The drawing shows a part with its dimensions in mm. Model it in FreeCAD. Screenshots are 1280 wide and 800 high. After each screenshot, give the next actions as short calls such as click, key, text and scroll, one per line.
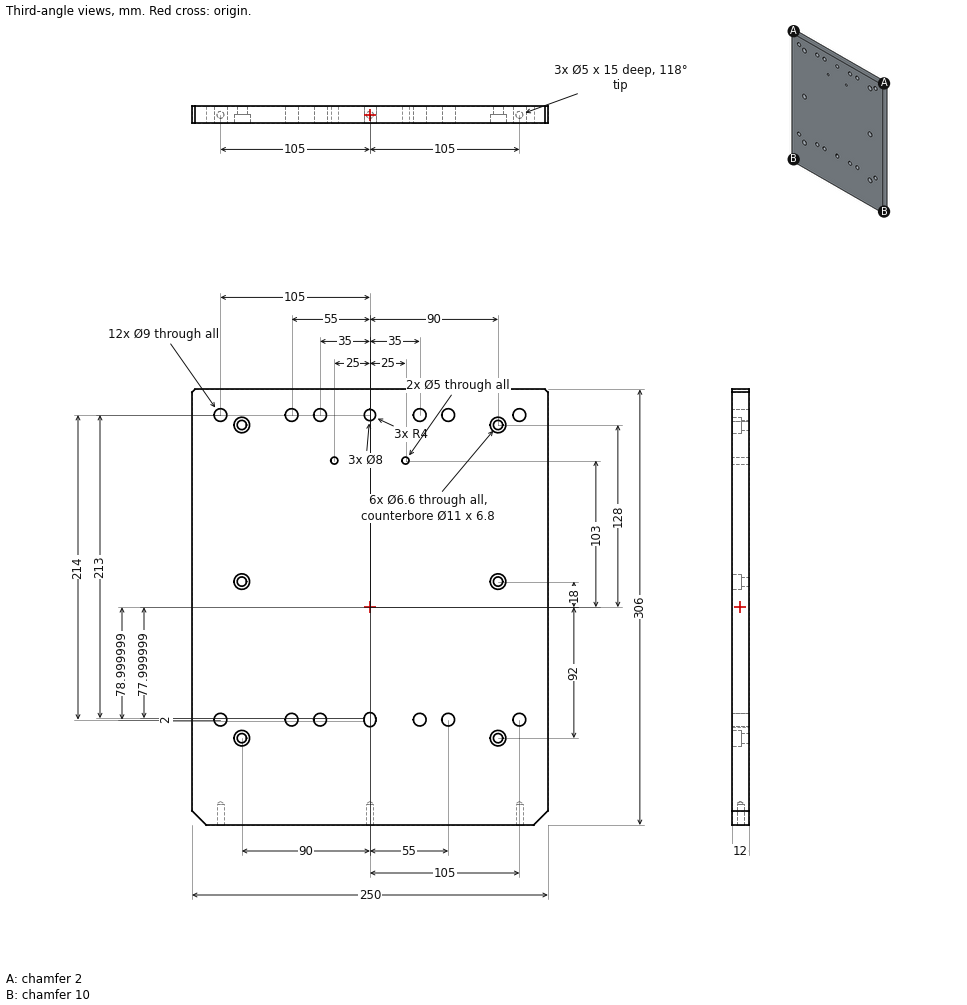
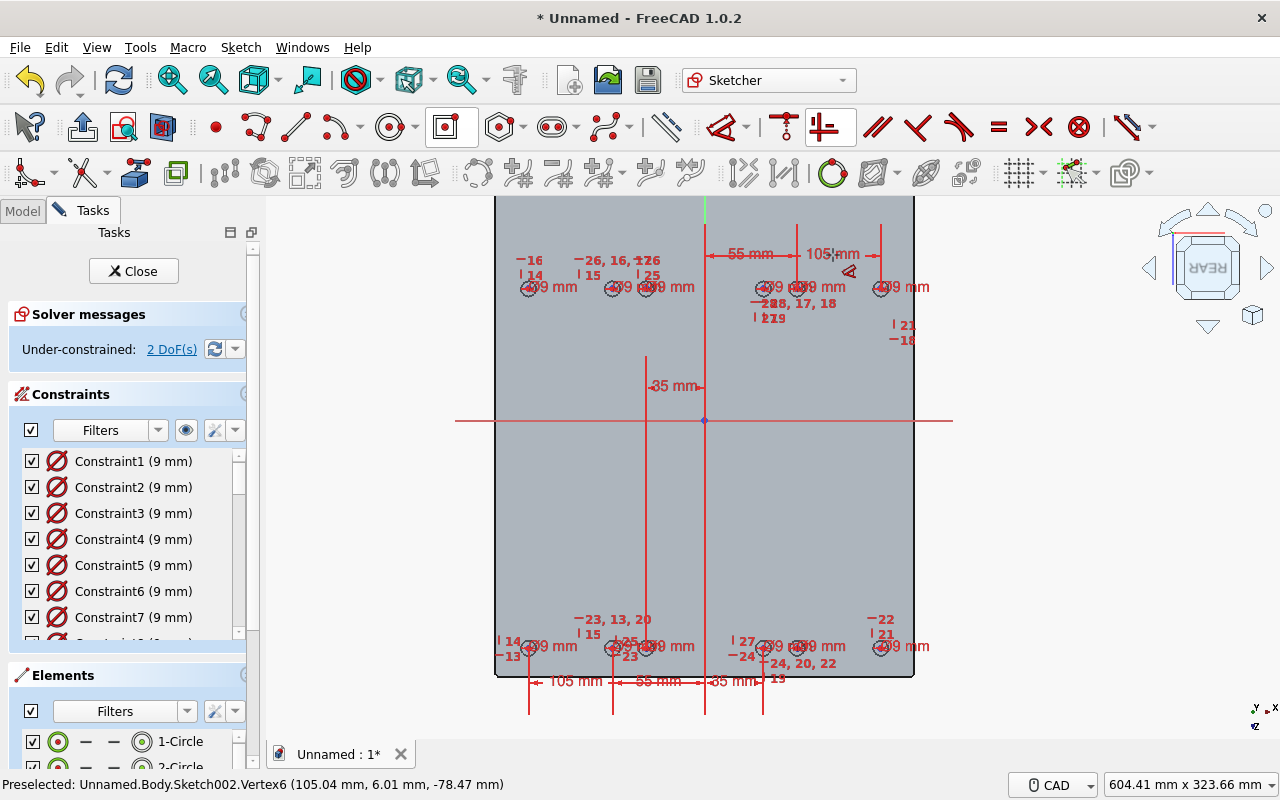
click(529, 648)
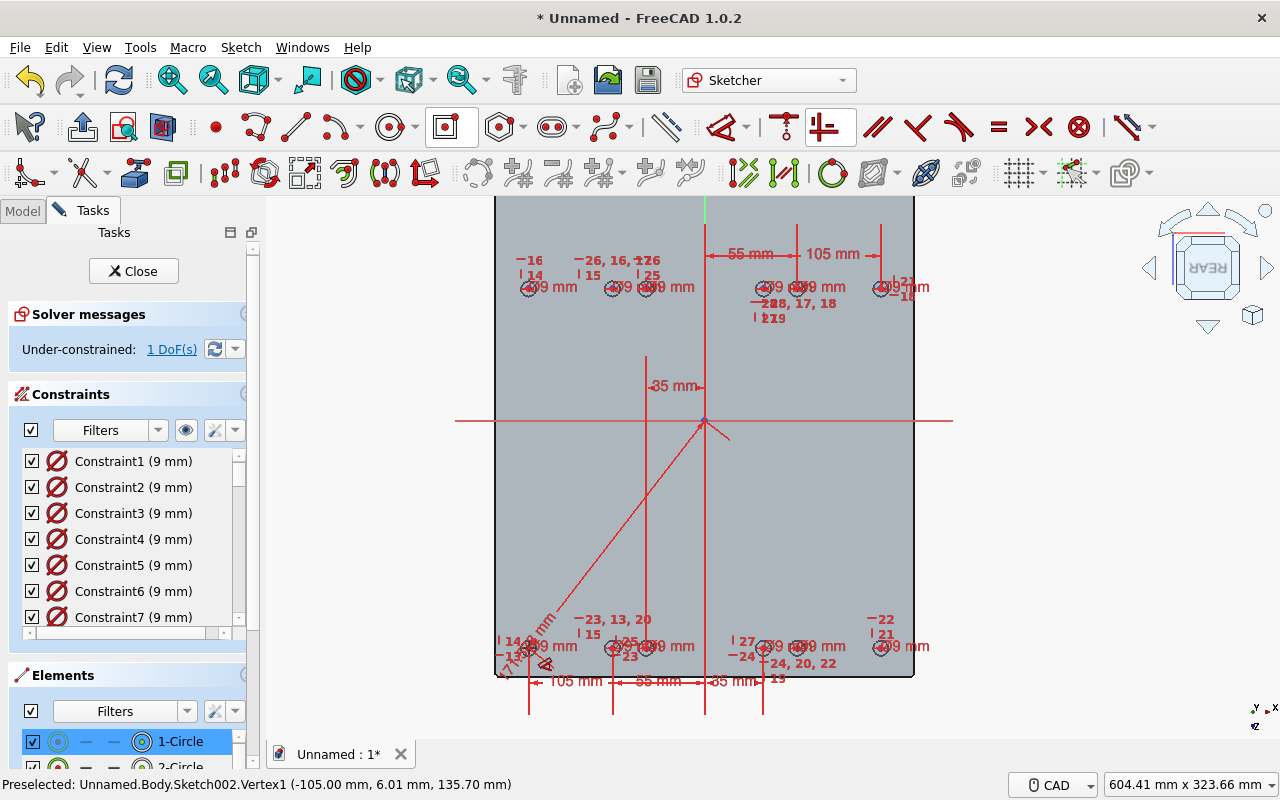
click(529, 289)
click(495, 469)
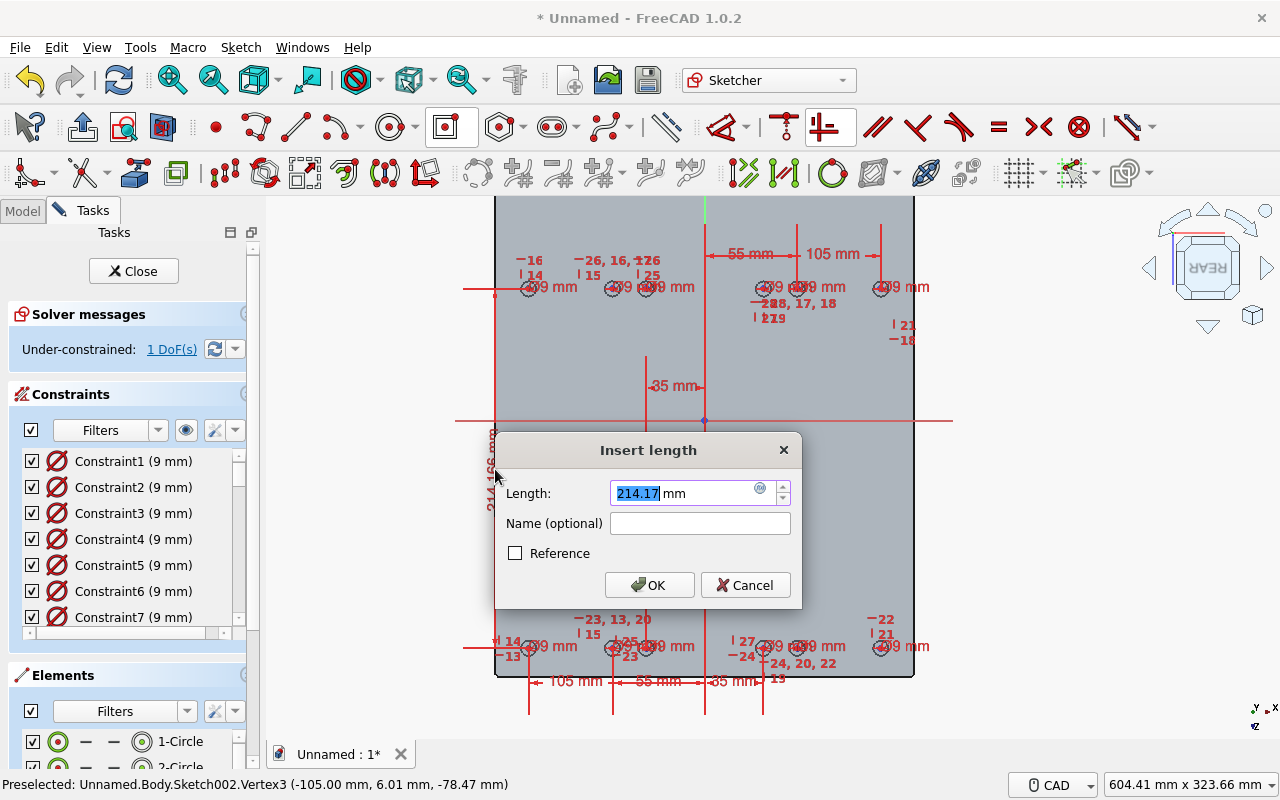
text(214)
key(Return)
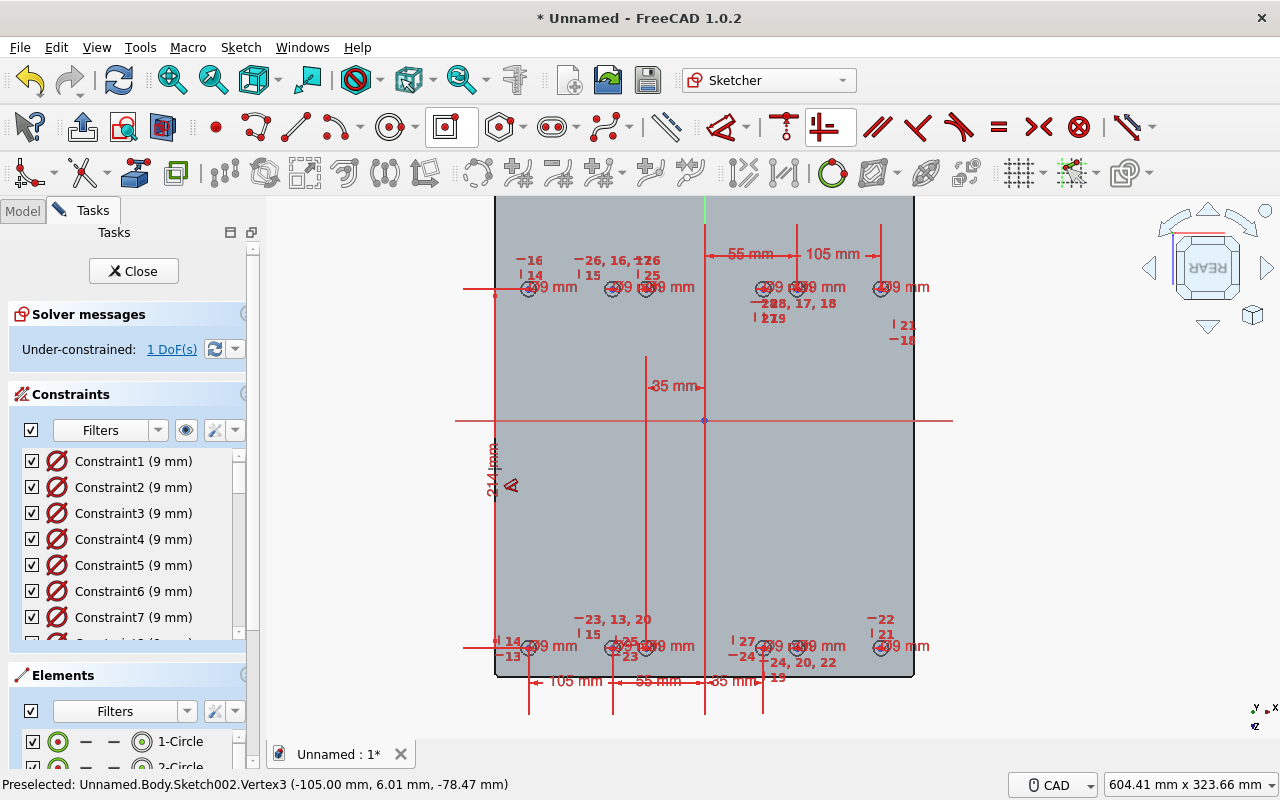
click(529, 289)
click(495, 355)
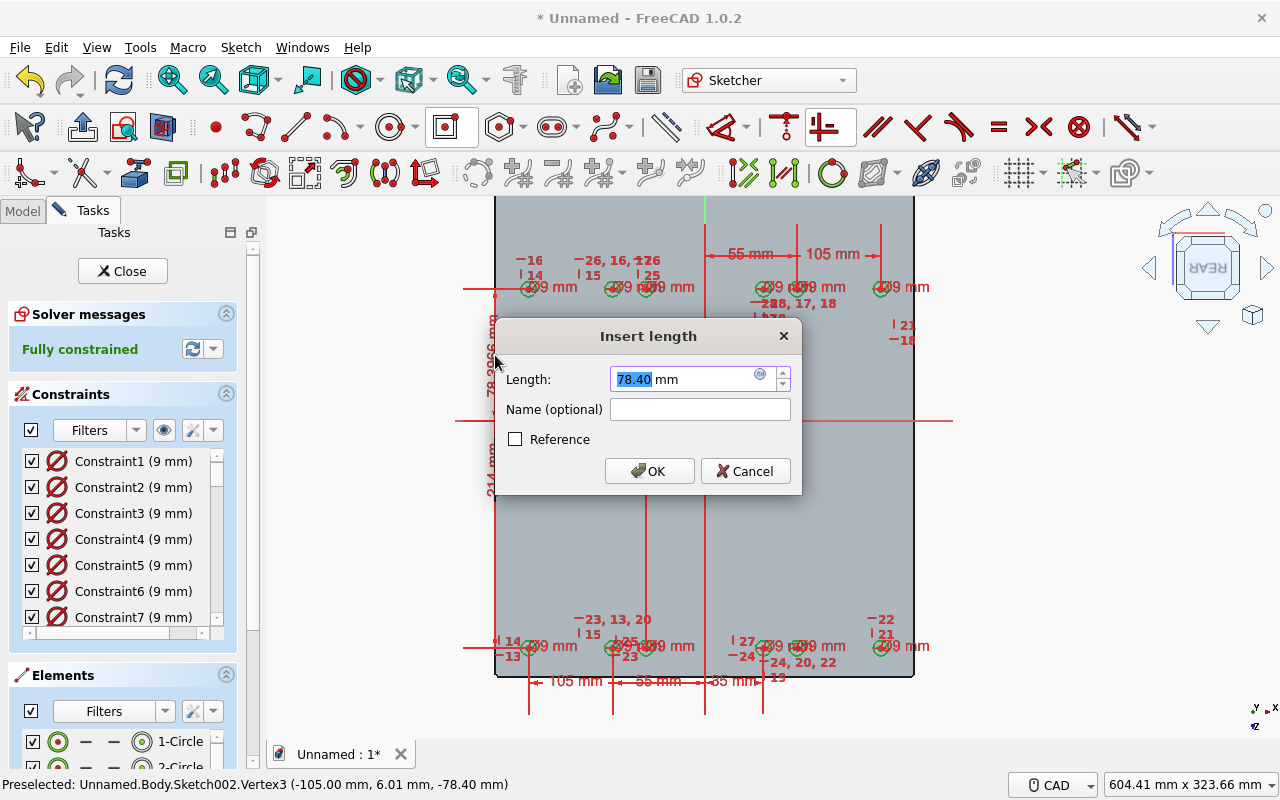
text(78.999999)
key(Return)
key(Escape)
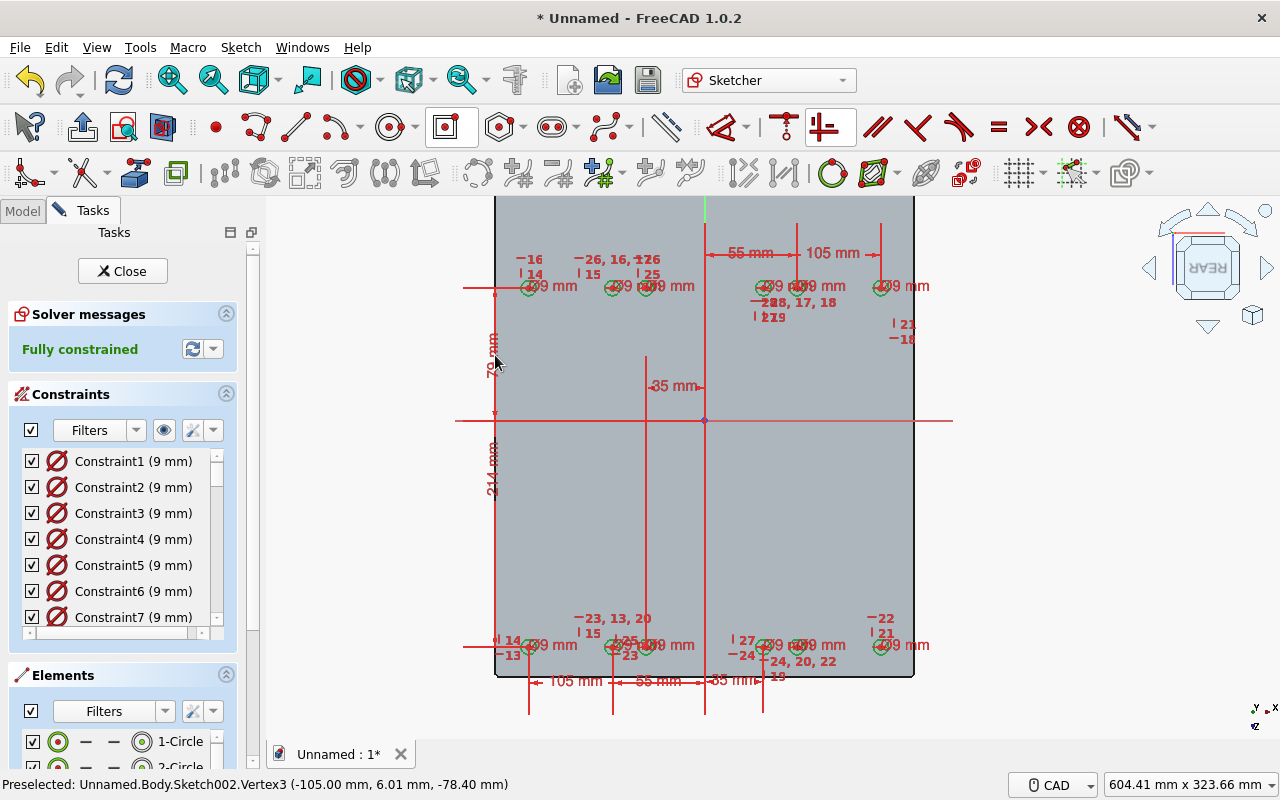
click(123, 271)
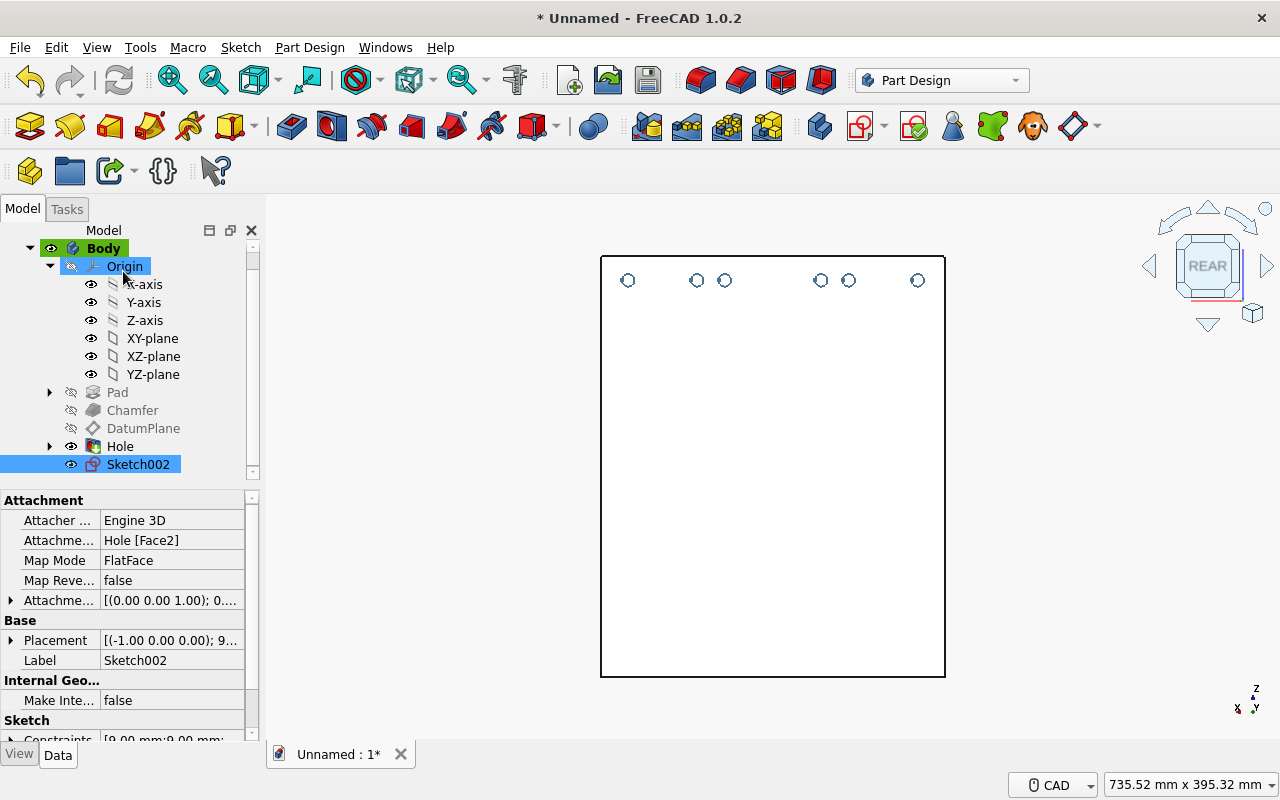
click(332, 126)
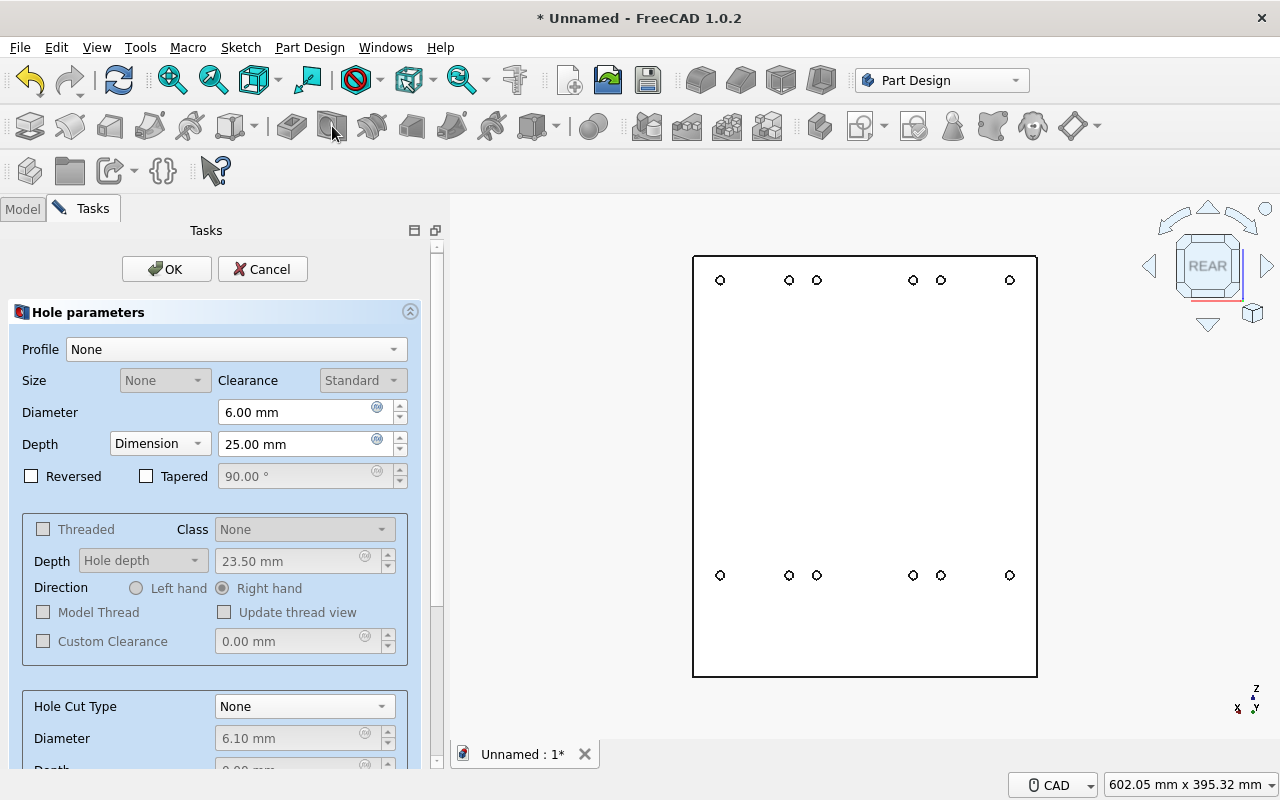
triple_click(305, 412)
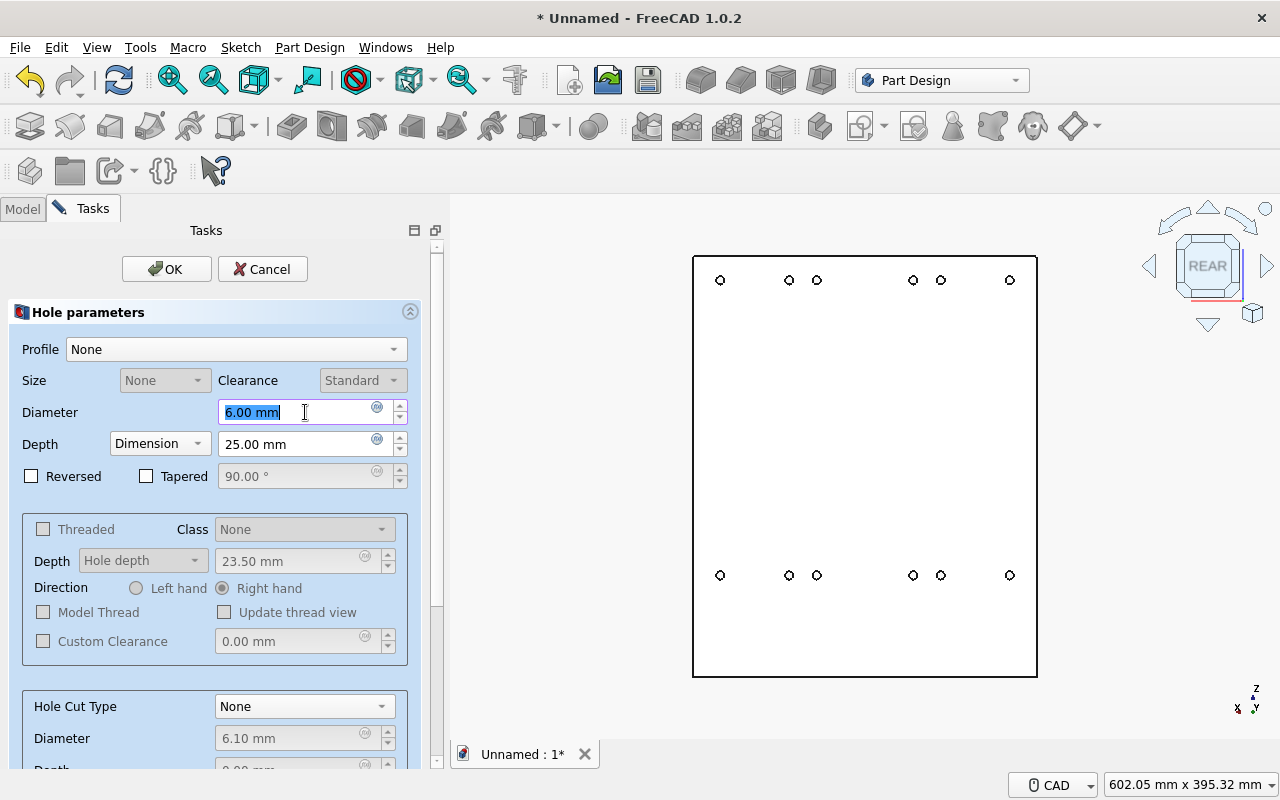
text(9)
key(Tab)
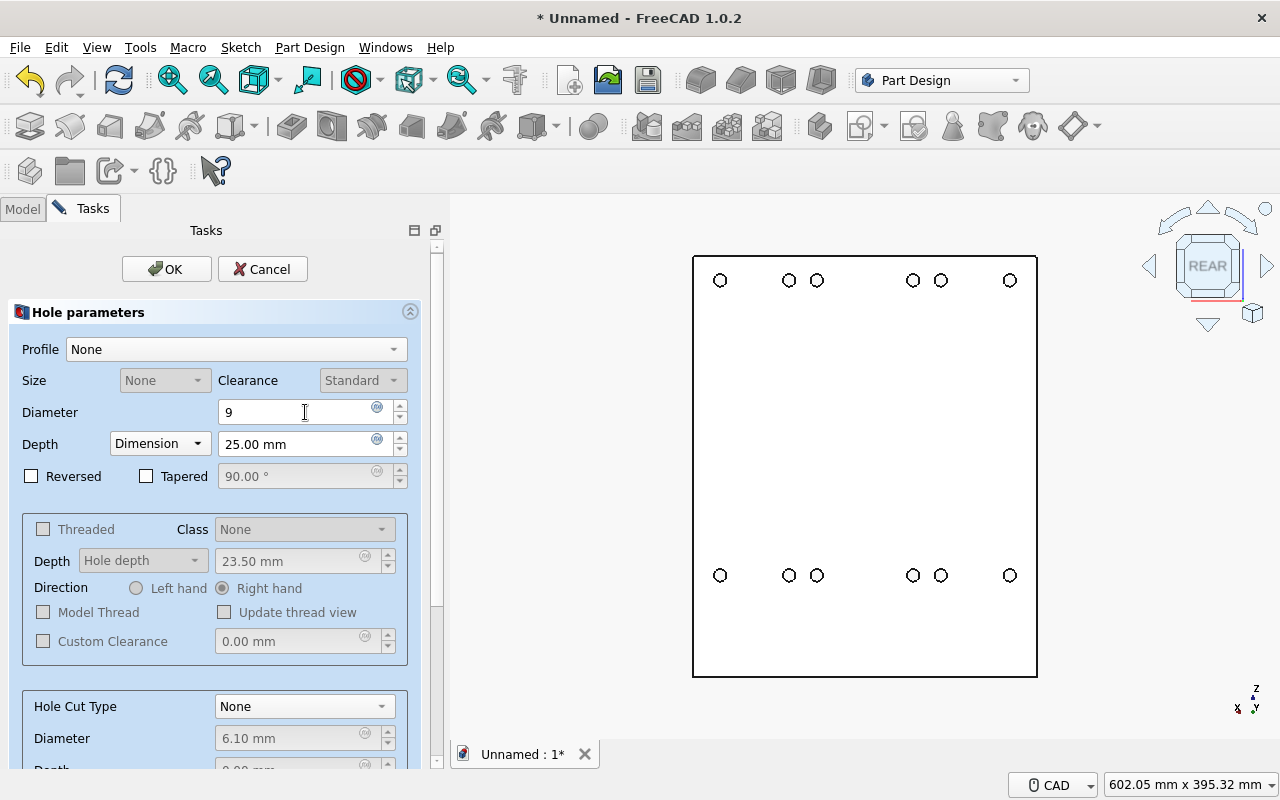
click(161, 444)